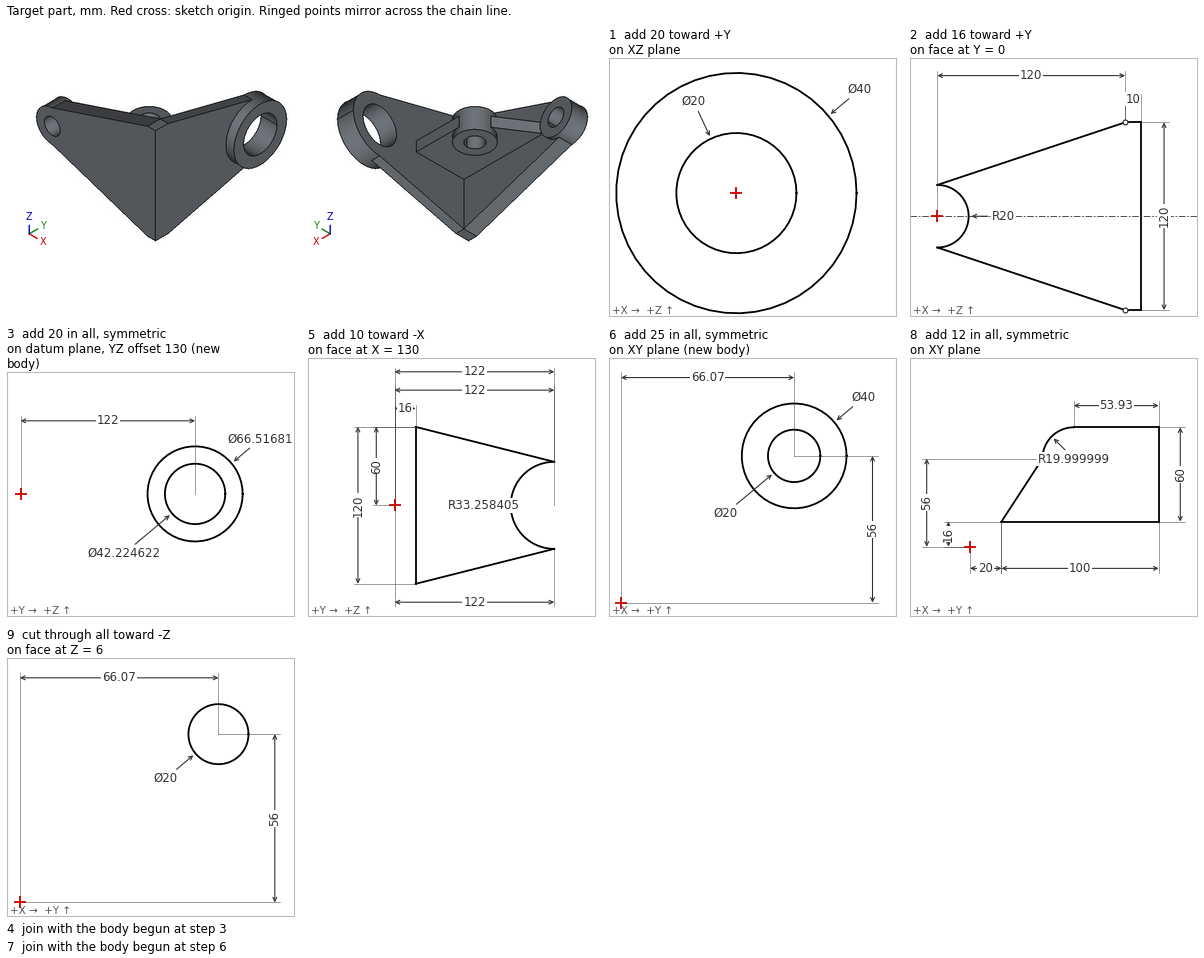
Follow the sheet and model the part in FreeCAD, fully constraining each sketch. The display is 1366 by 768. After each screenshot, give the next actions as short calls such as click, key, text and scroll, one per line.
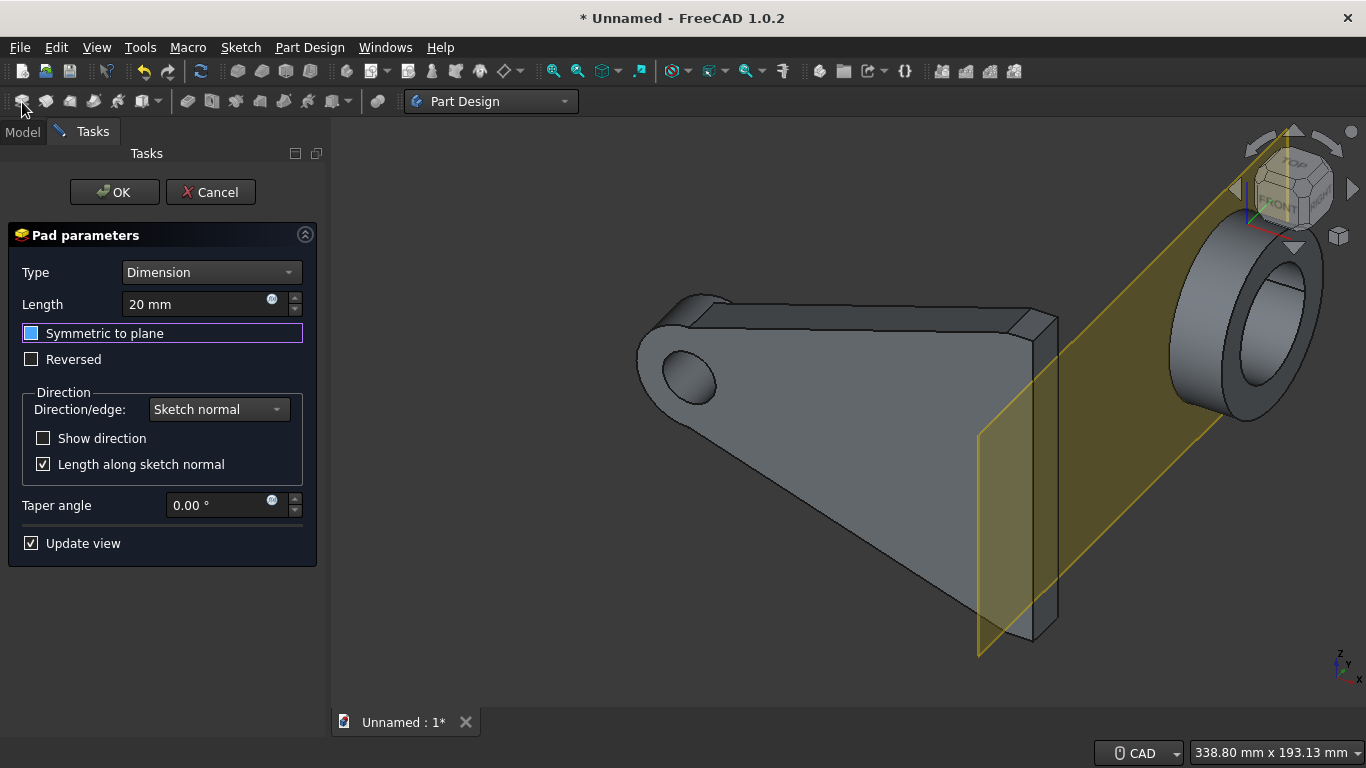
click(30, 333)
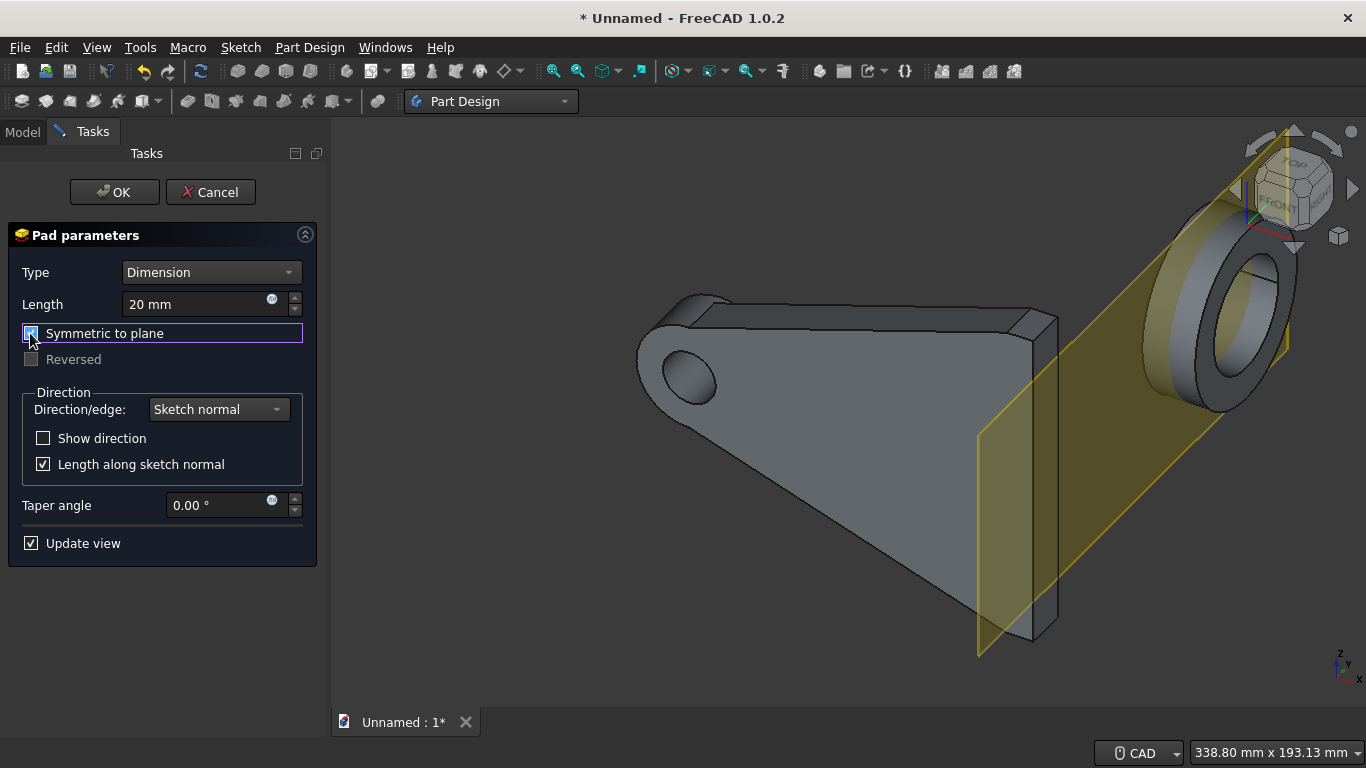
click(115, 192)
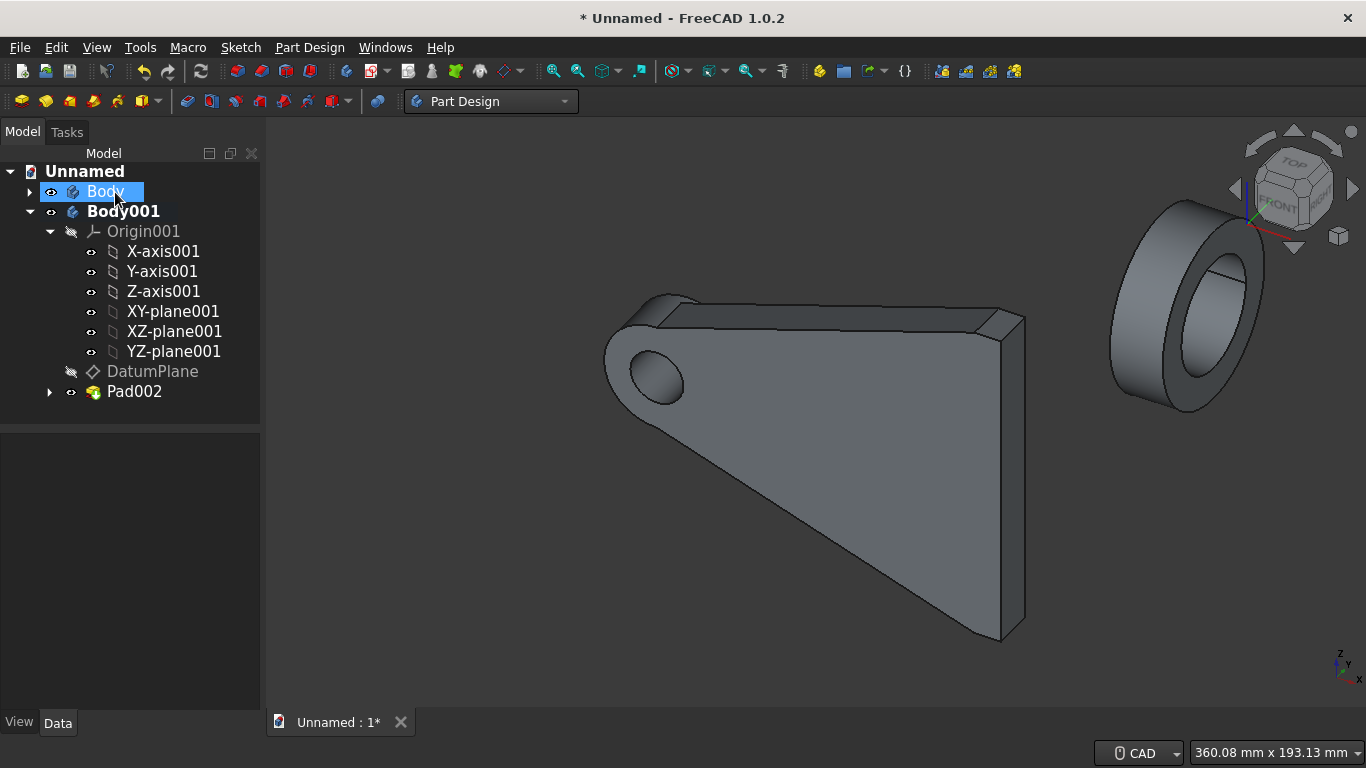
double_click(96, 192)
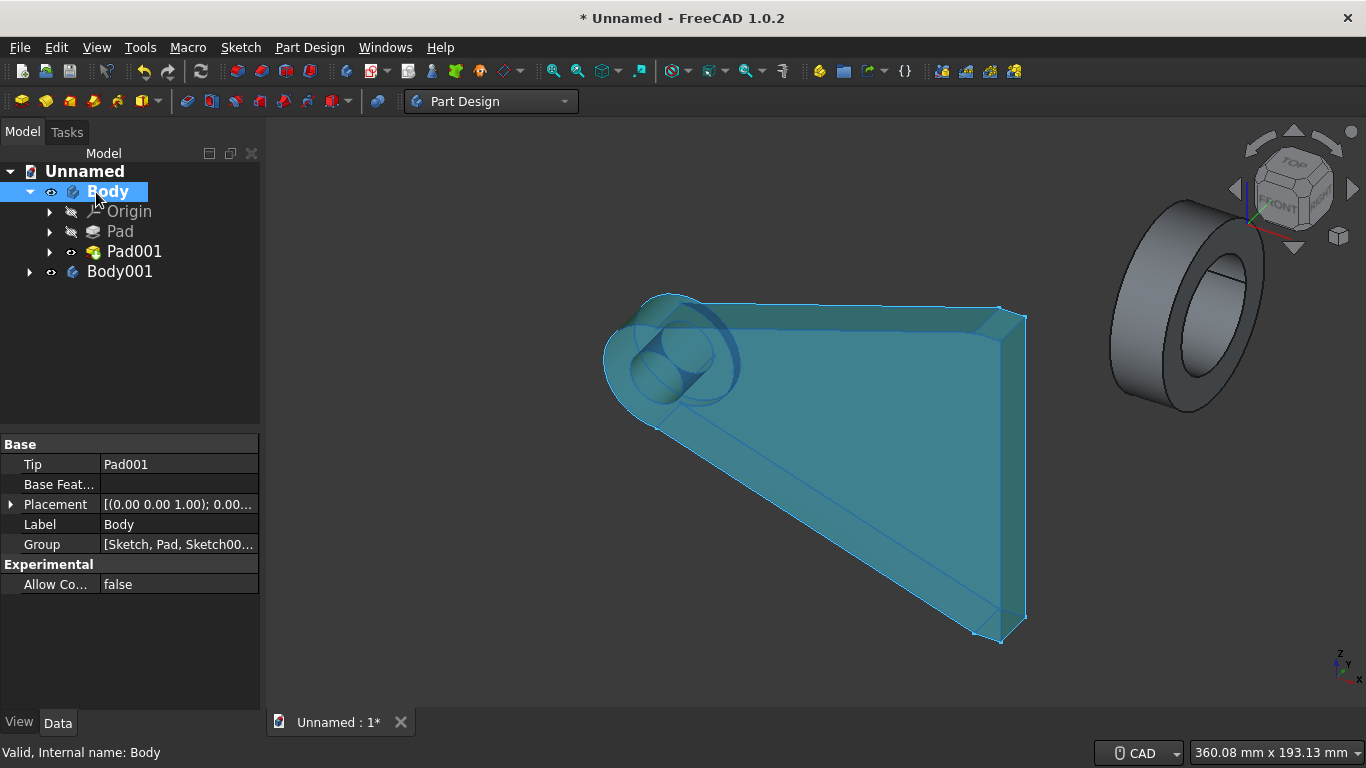
click(96, 192)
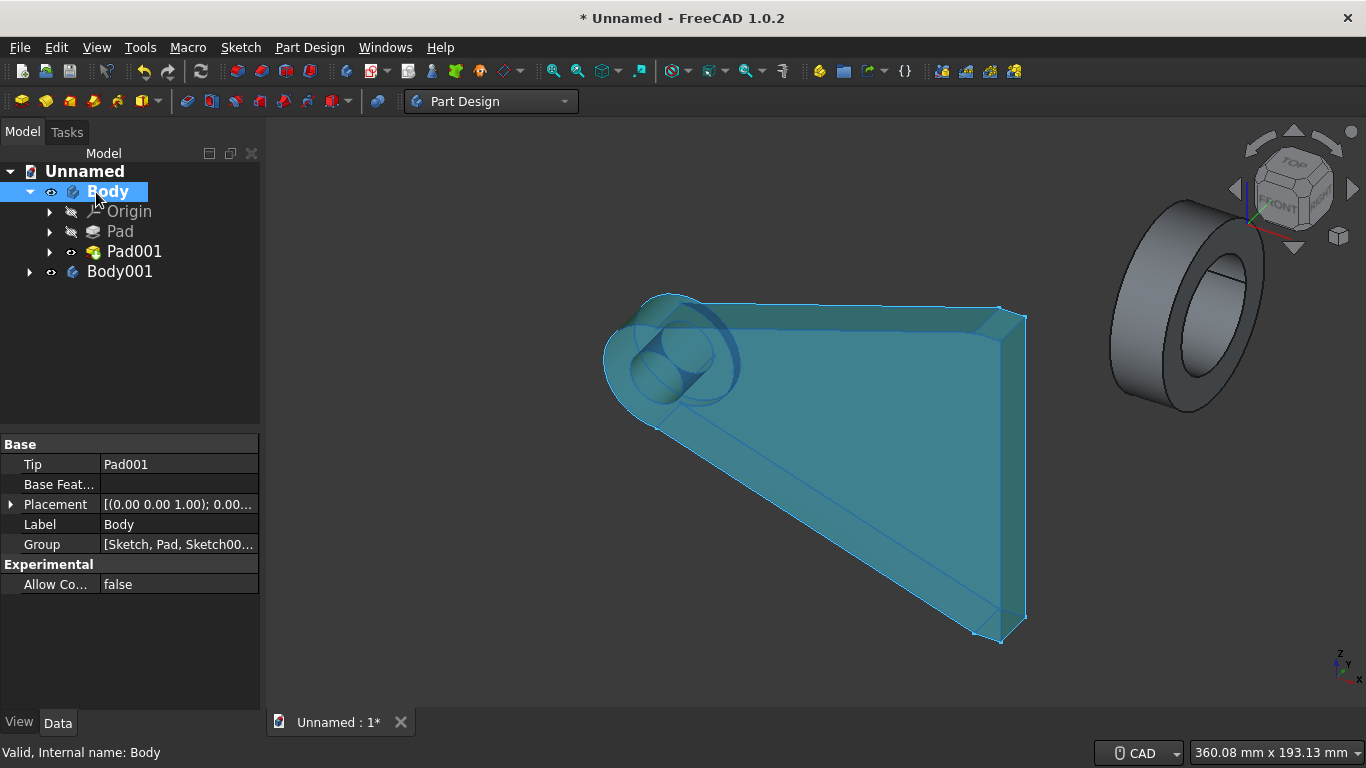
click(146, 584)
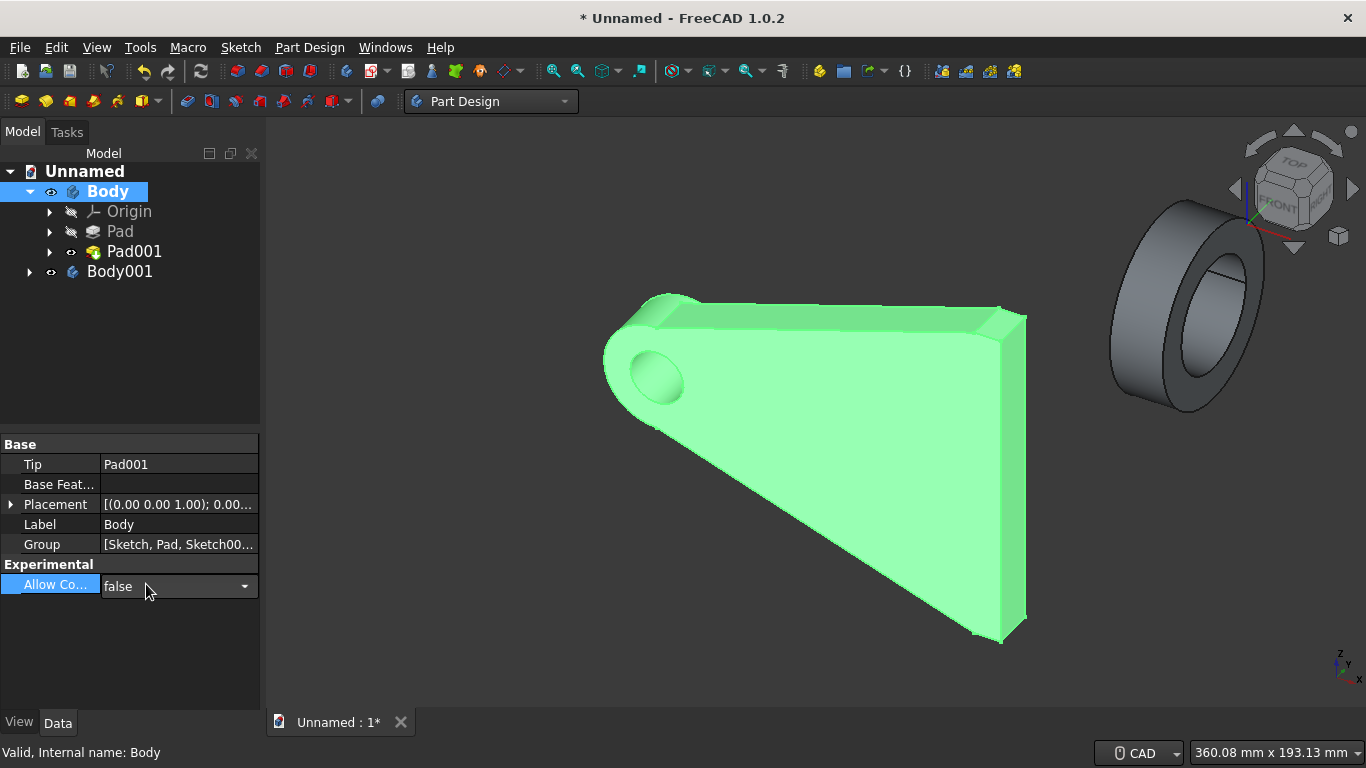
click(146, 584)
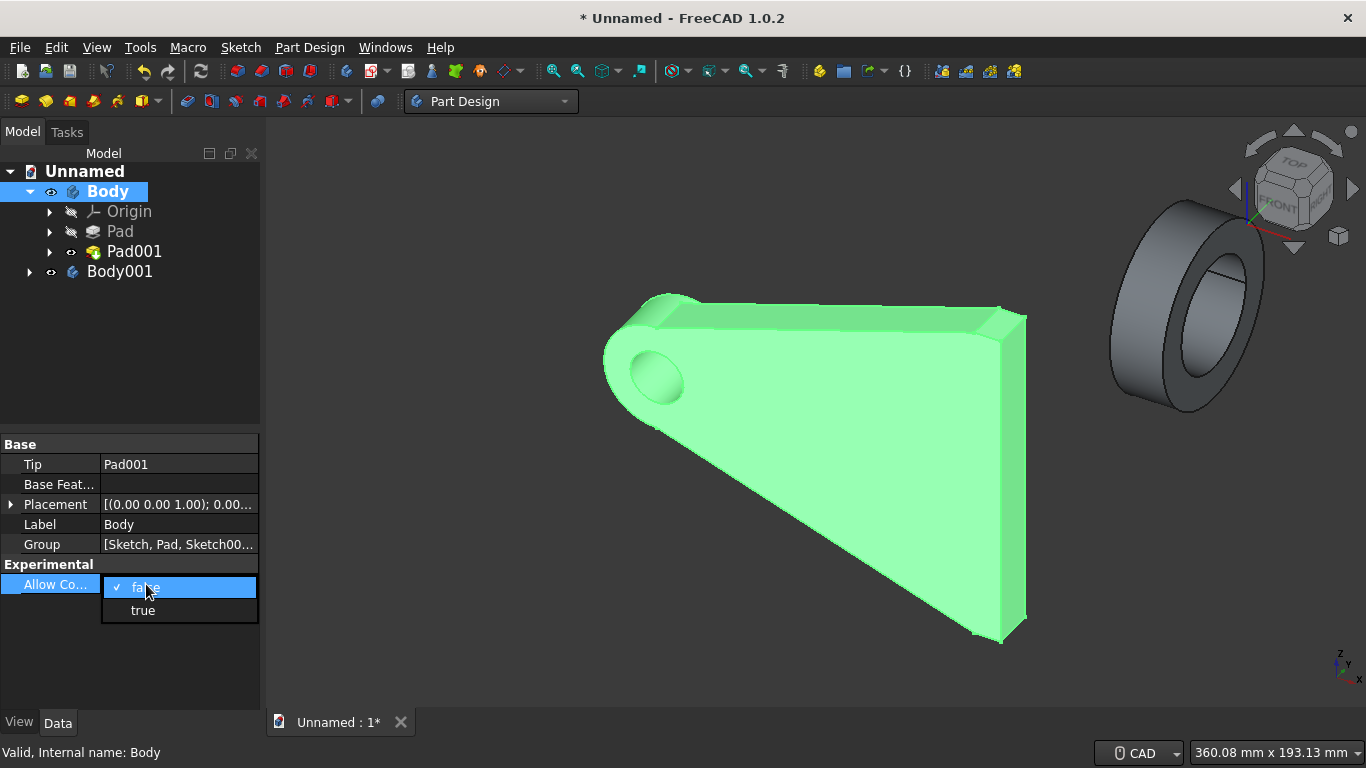
click(179, 610)
key(Return)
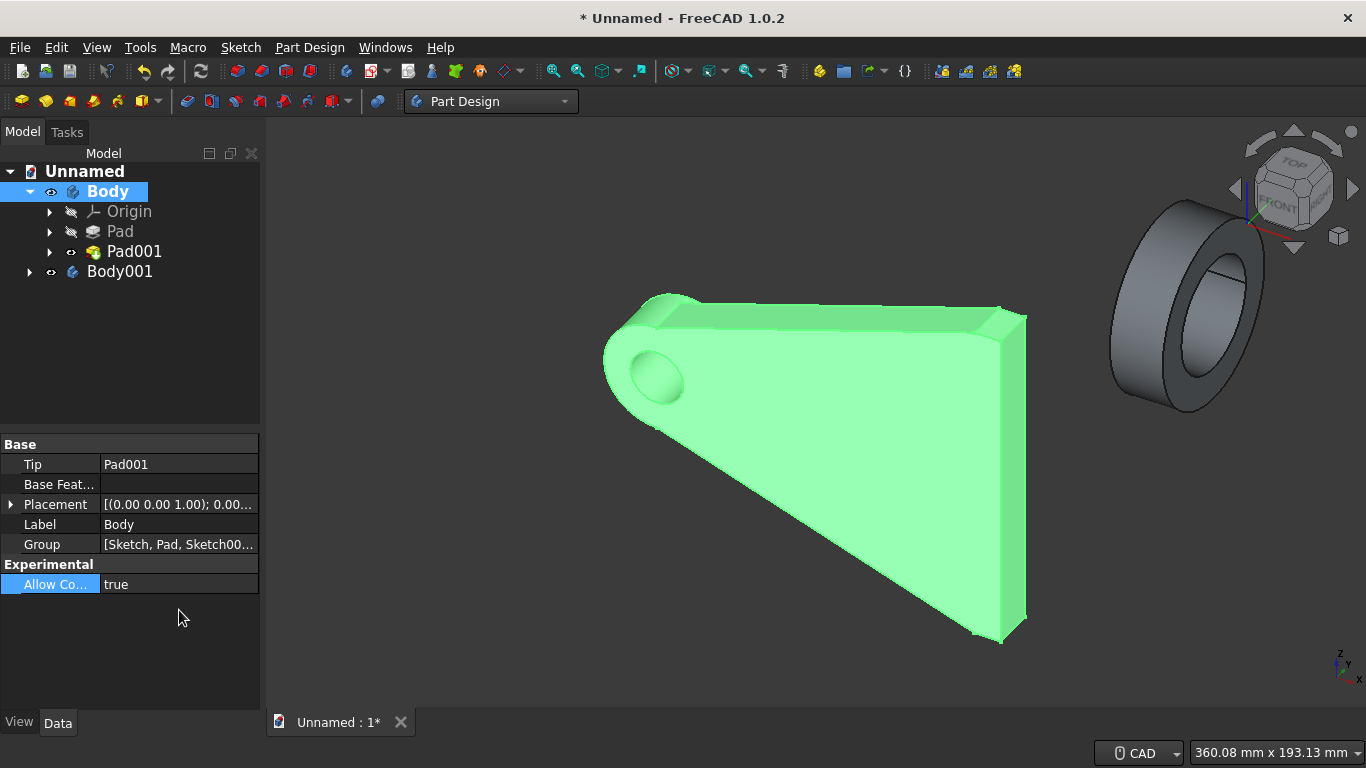
click(96, 272)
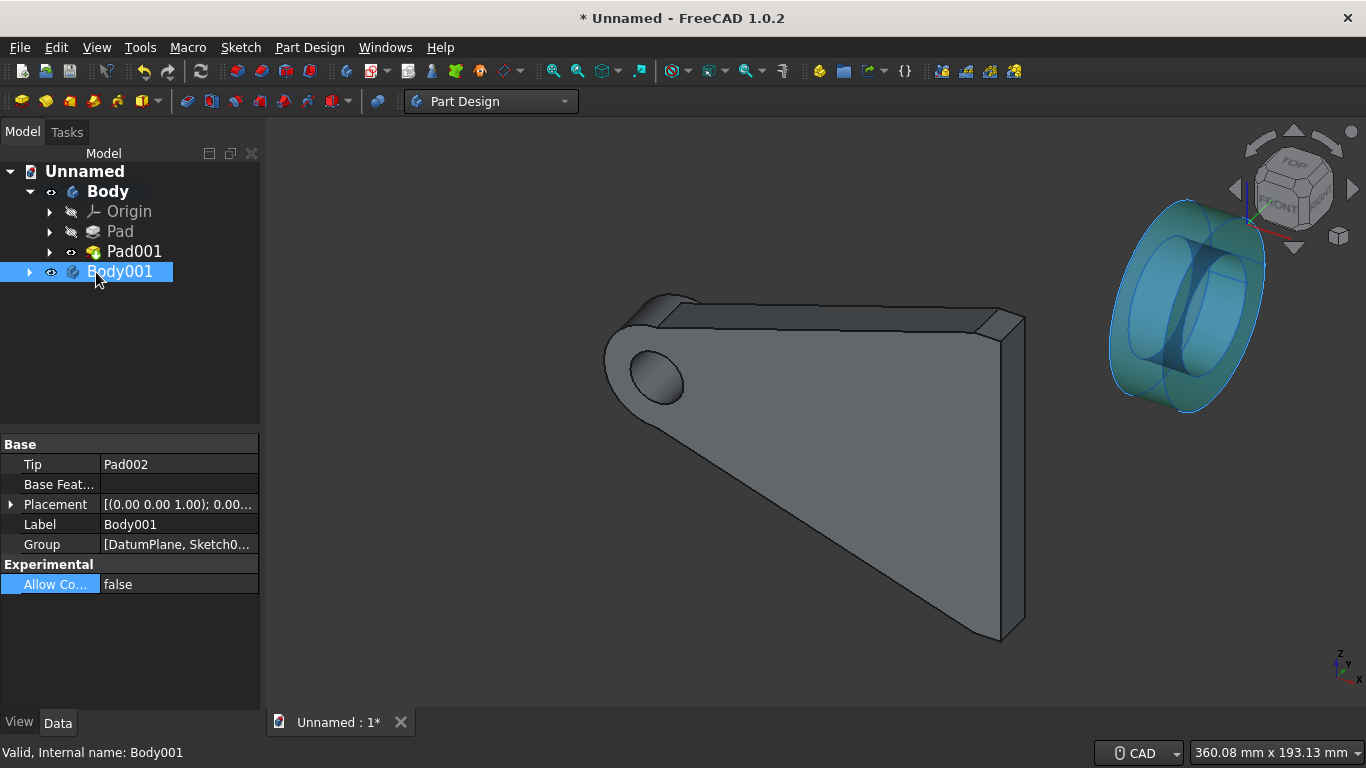
click(378, 102)